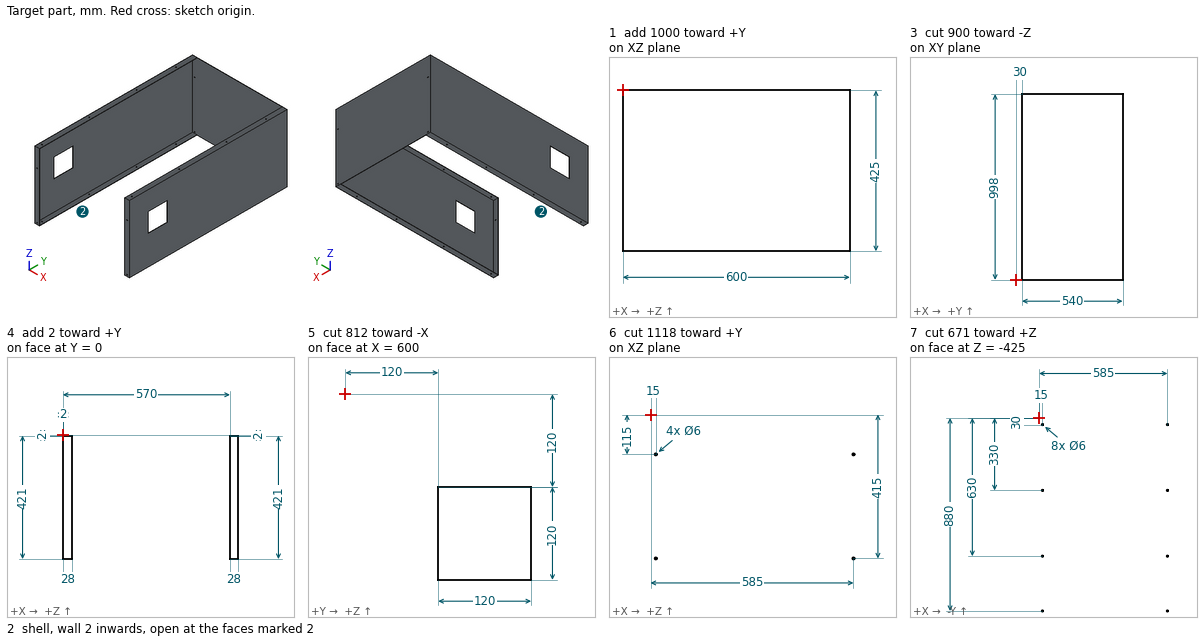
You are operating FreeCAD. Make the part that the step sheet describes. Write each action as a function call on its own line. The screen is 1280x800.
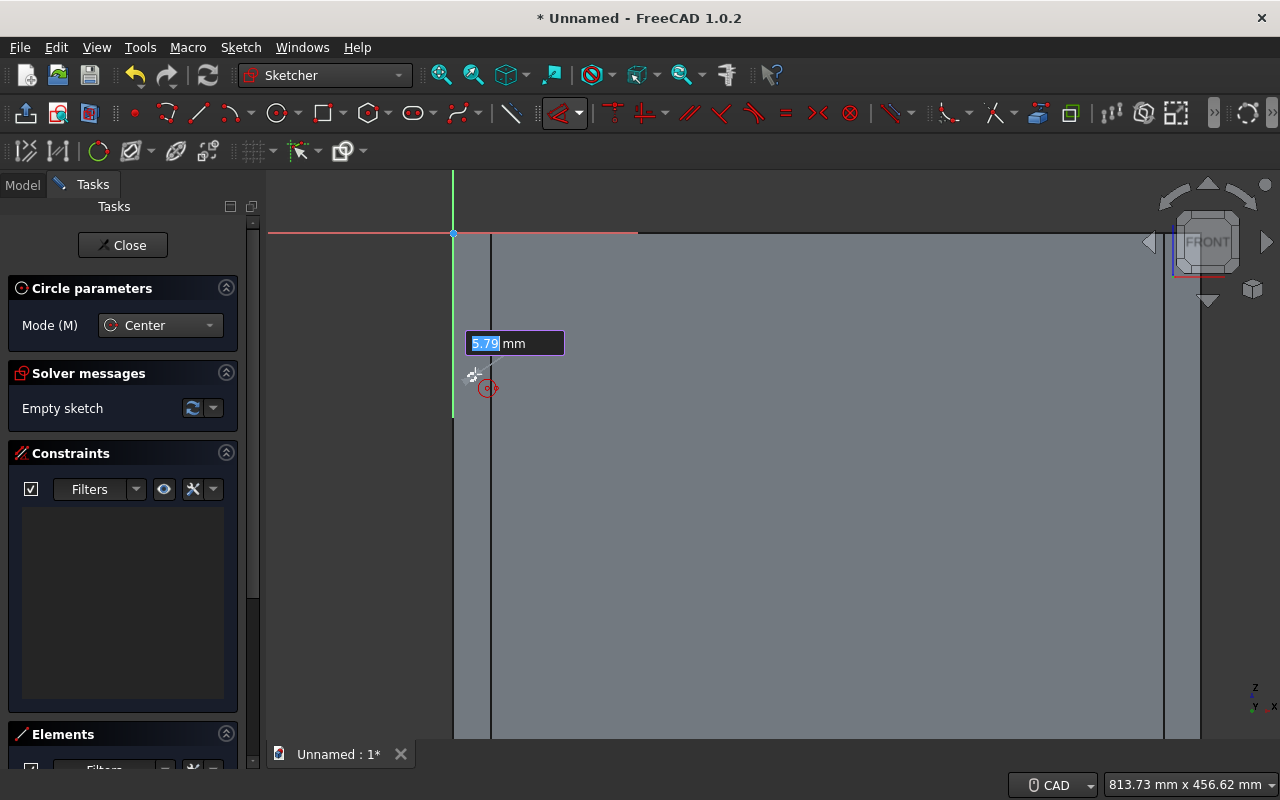
text(6)
key(Return)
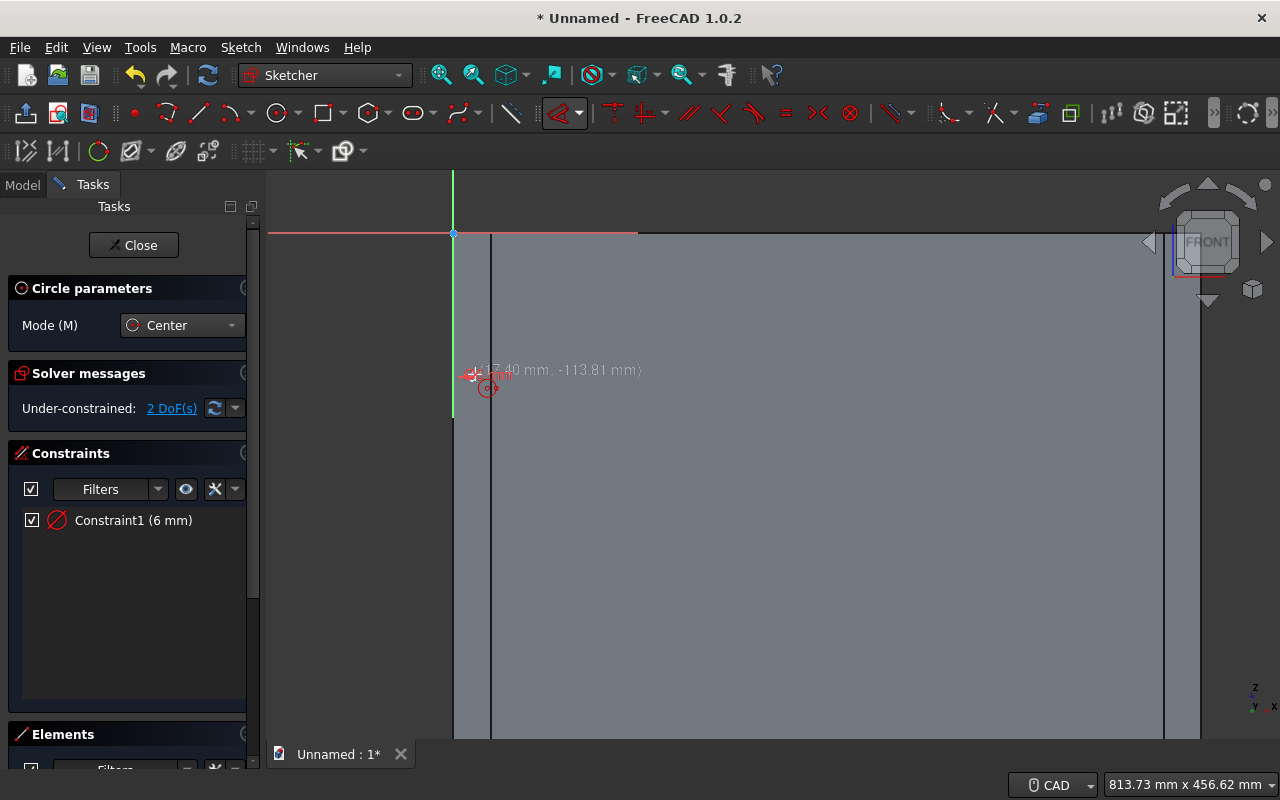
scroll(470, 375, down, 2)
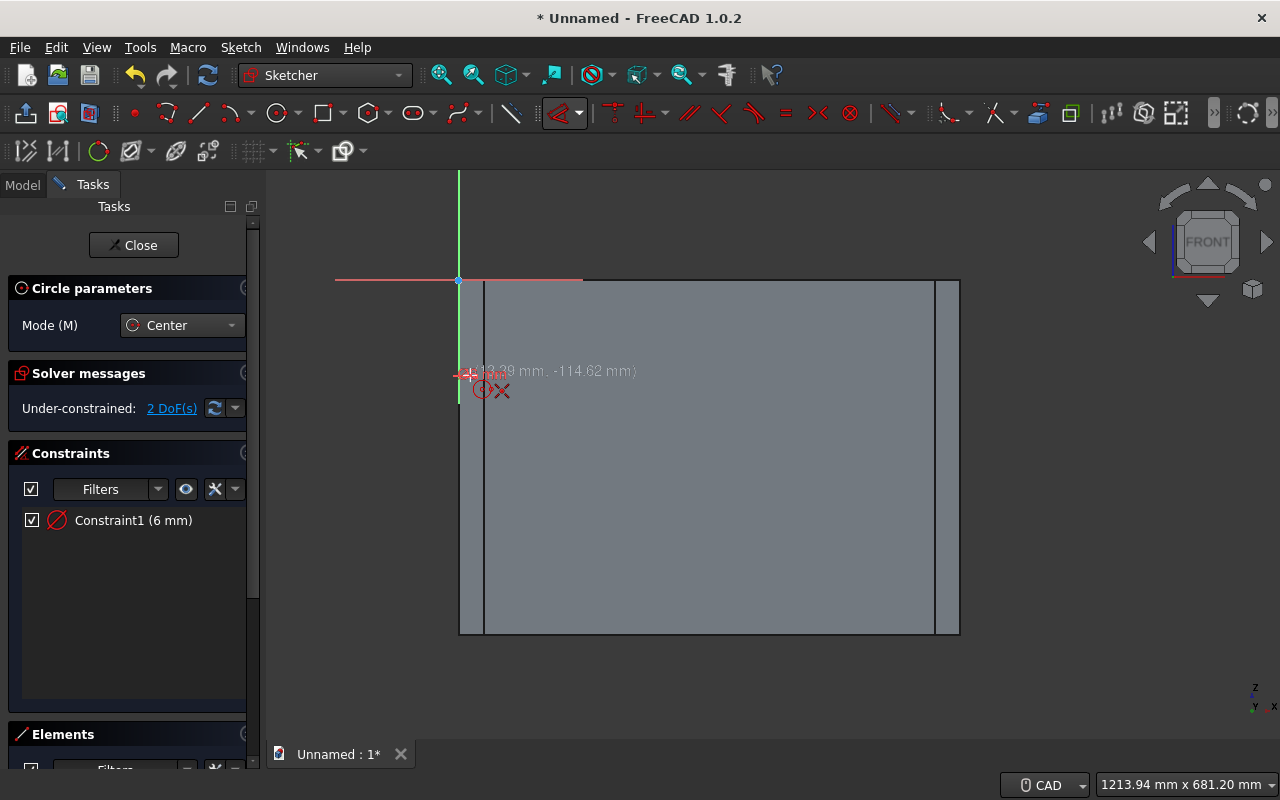
scroll(948, 627, up, 12)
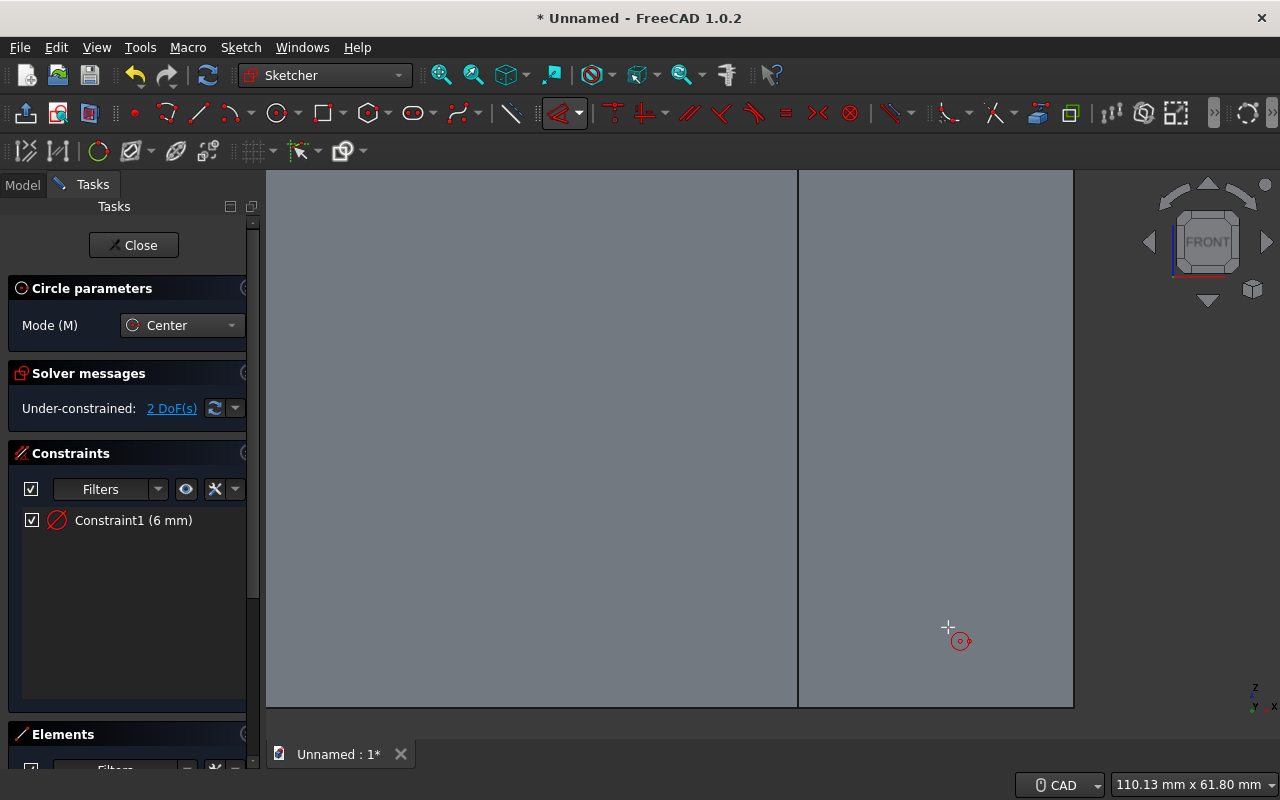
scroll(949, 628, down, 12)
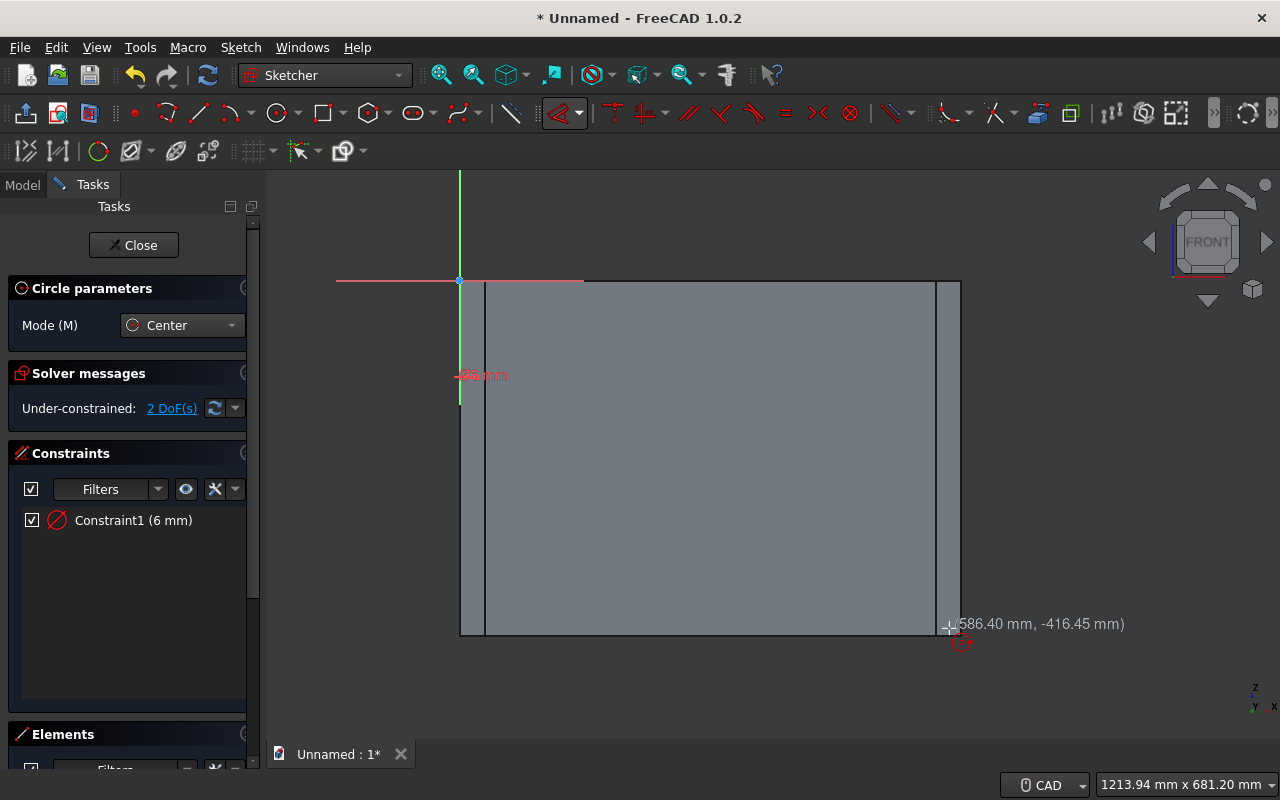
click(948, 628)
move(950, 626)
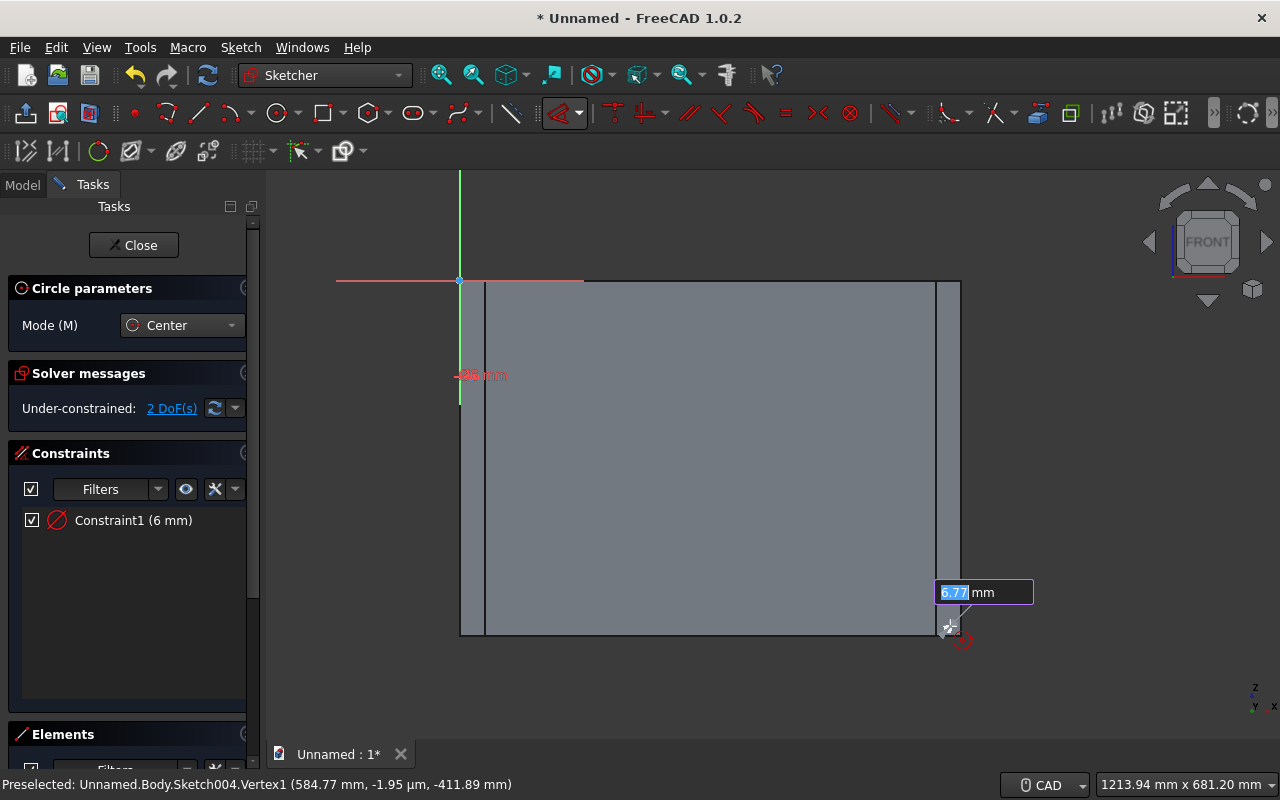
text(6)
key(Return)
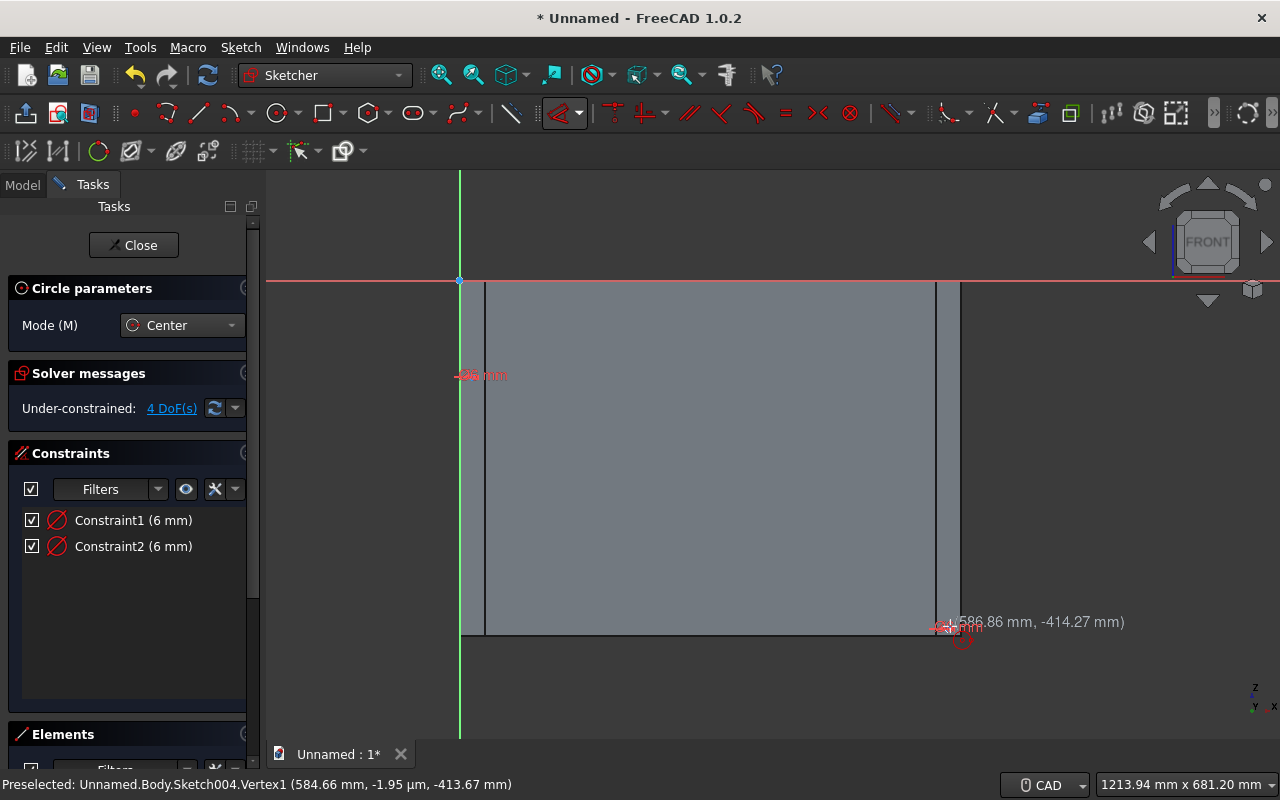
scroll(472, 628, up, 12)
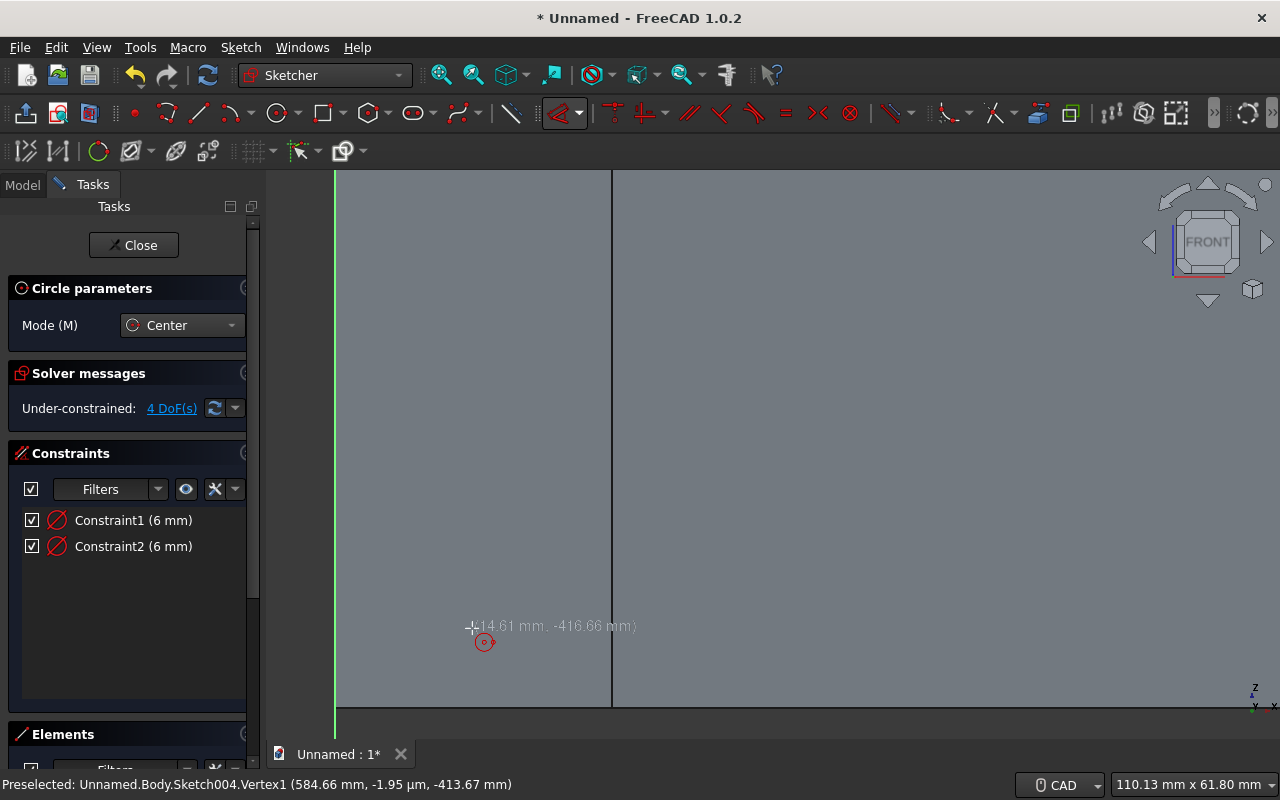
scroll(471, 628, down, 12)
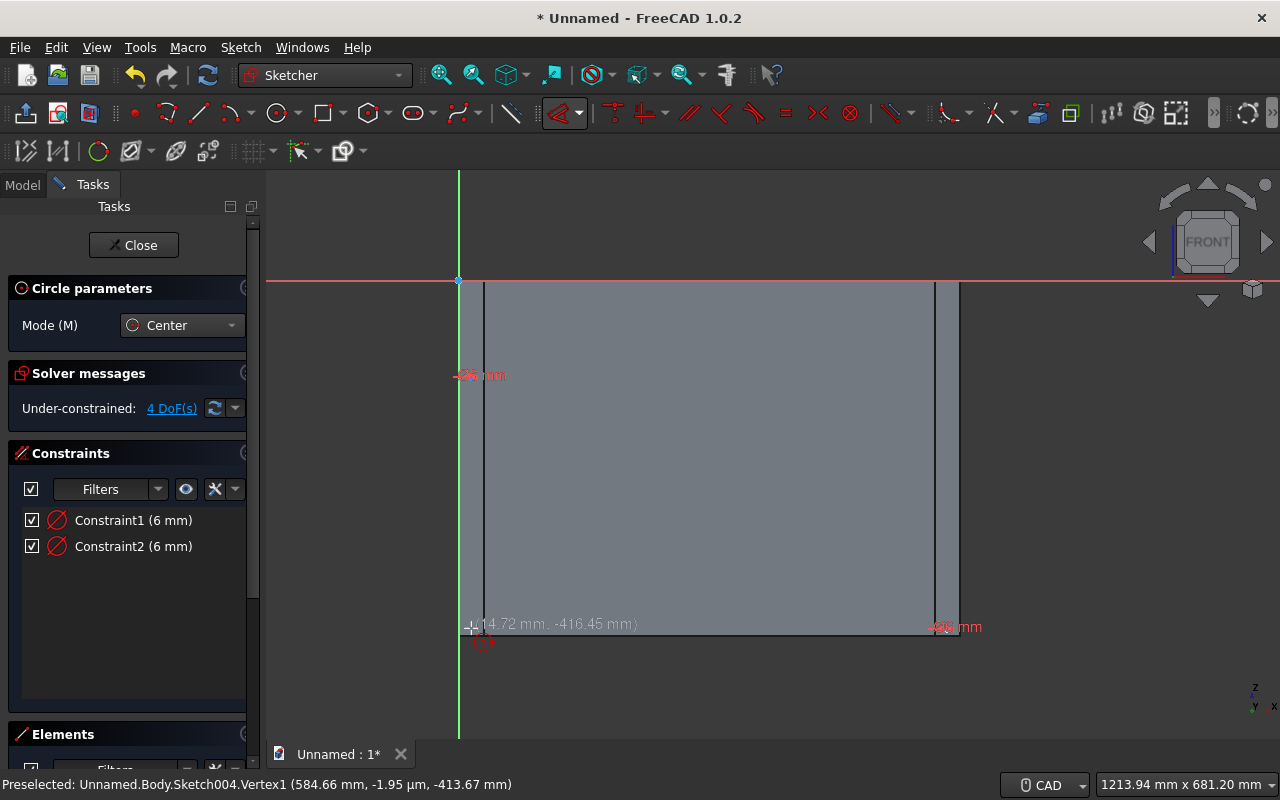
scroll(471, 628, up, 2)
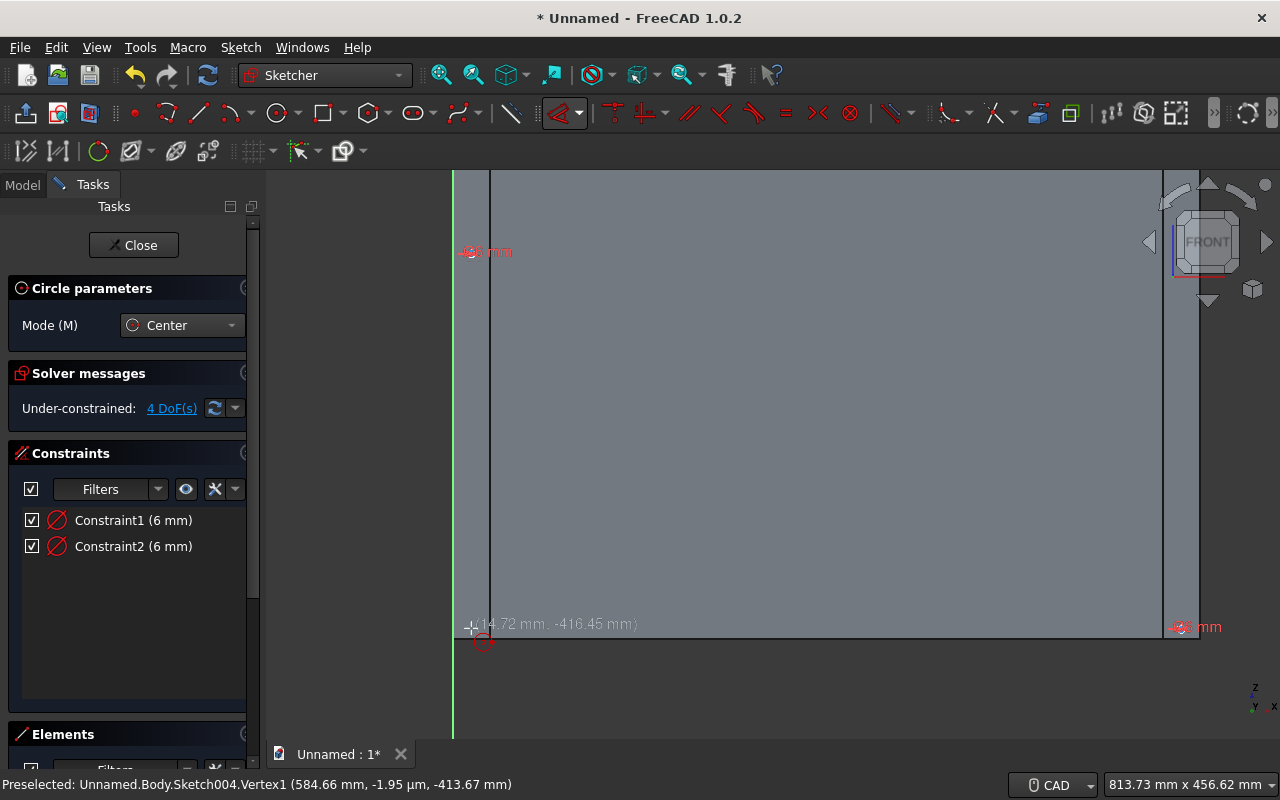
click(472, 627)
move(474, 624)